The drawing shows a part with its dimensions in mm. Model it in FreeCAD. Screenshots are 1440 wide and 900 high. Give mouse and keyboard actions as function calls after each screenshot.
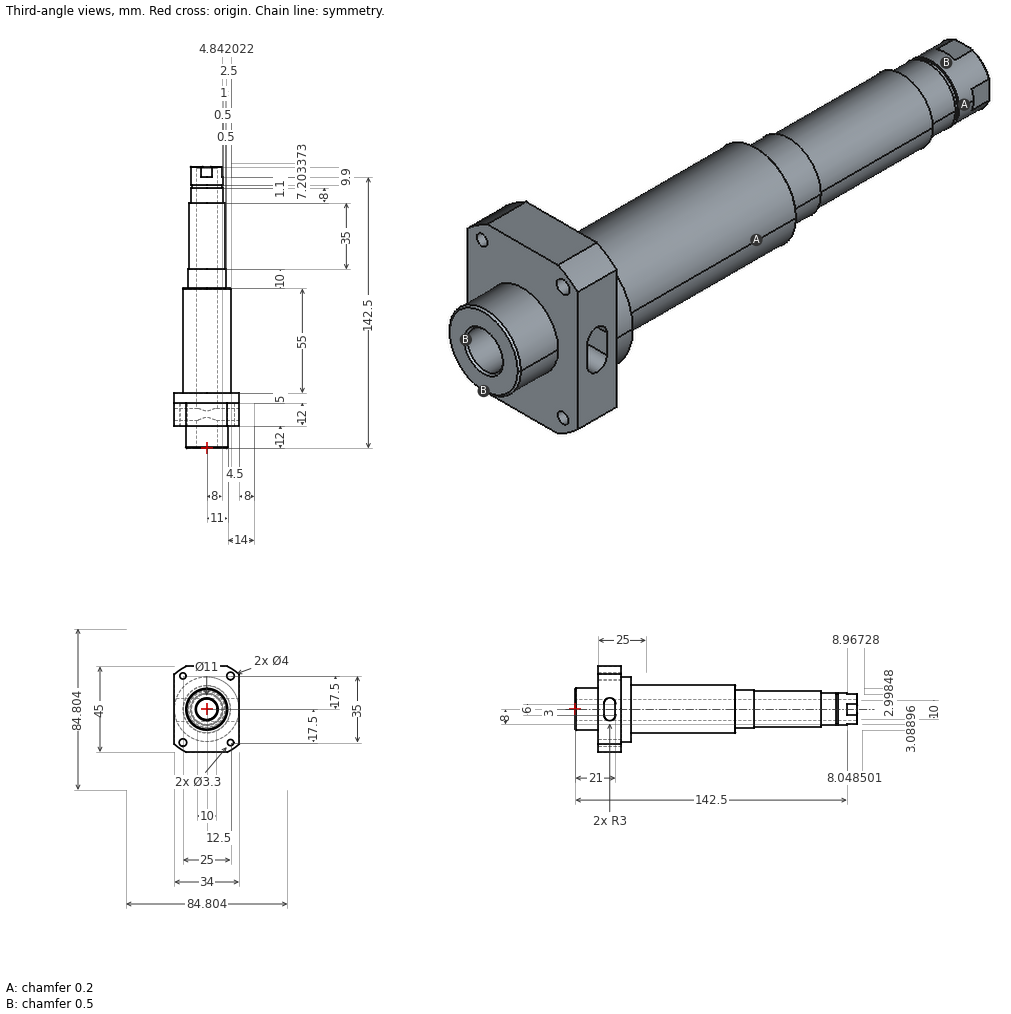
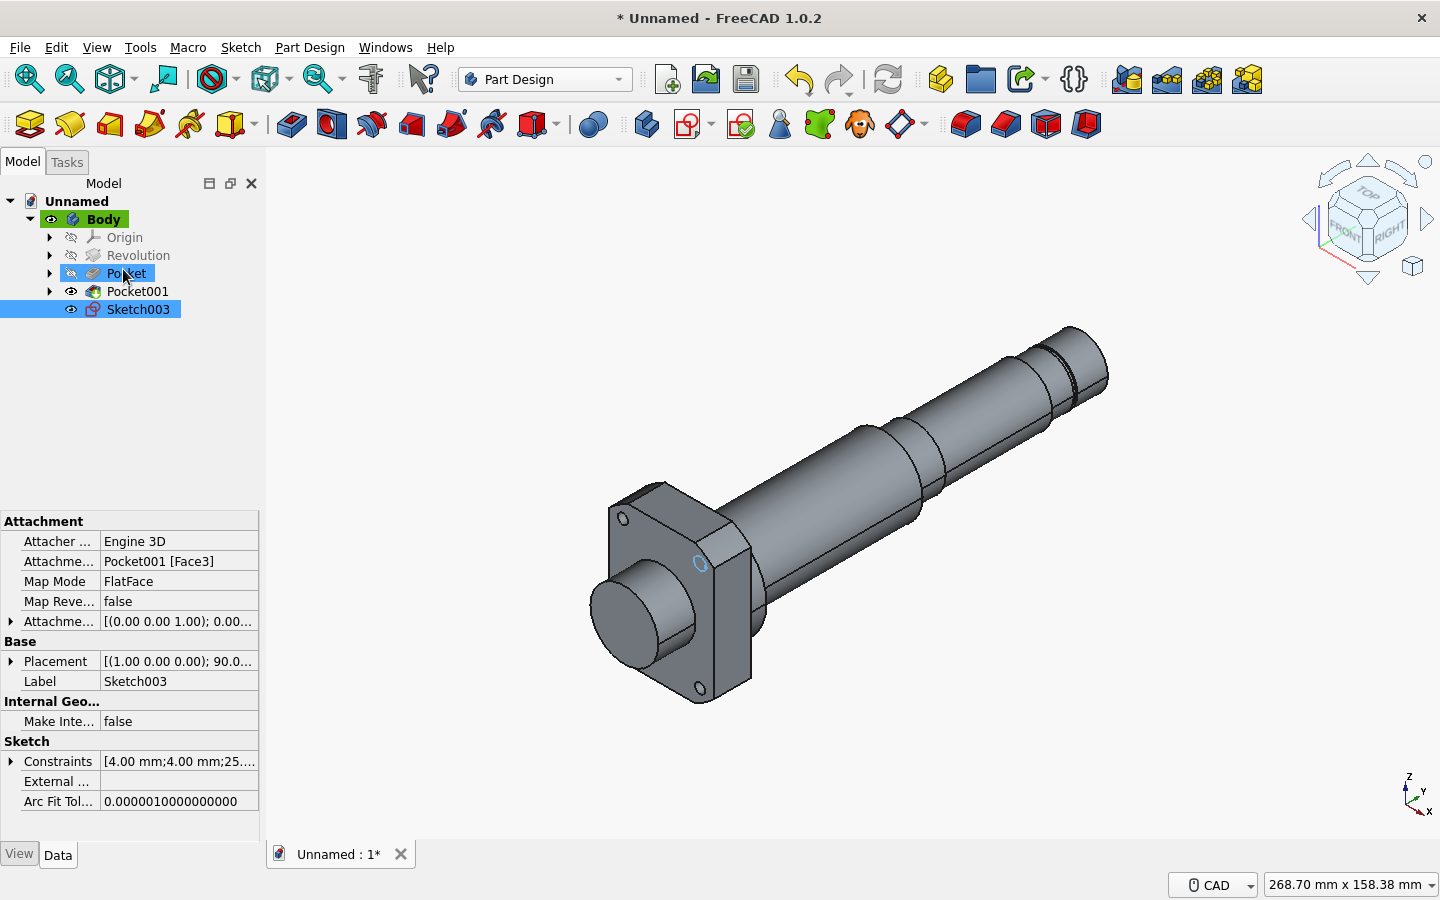
click(292, 124)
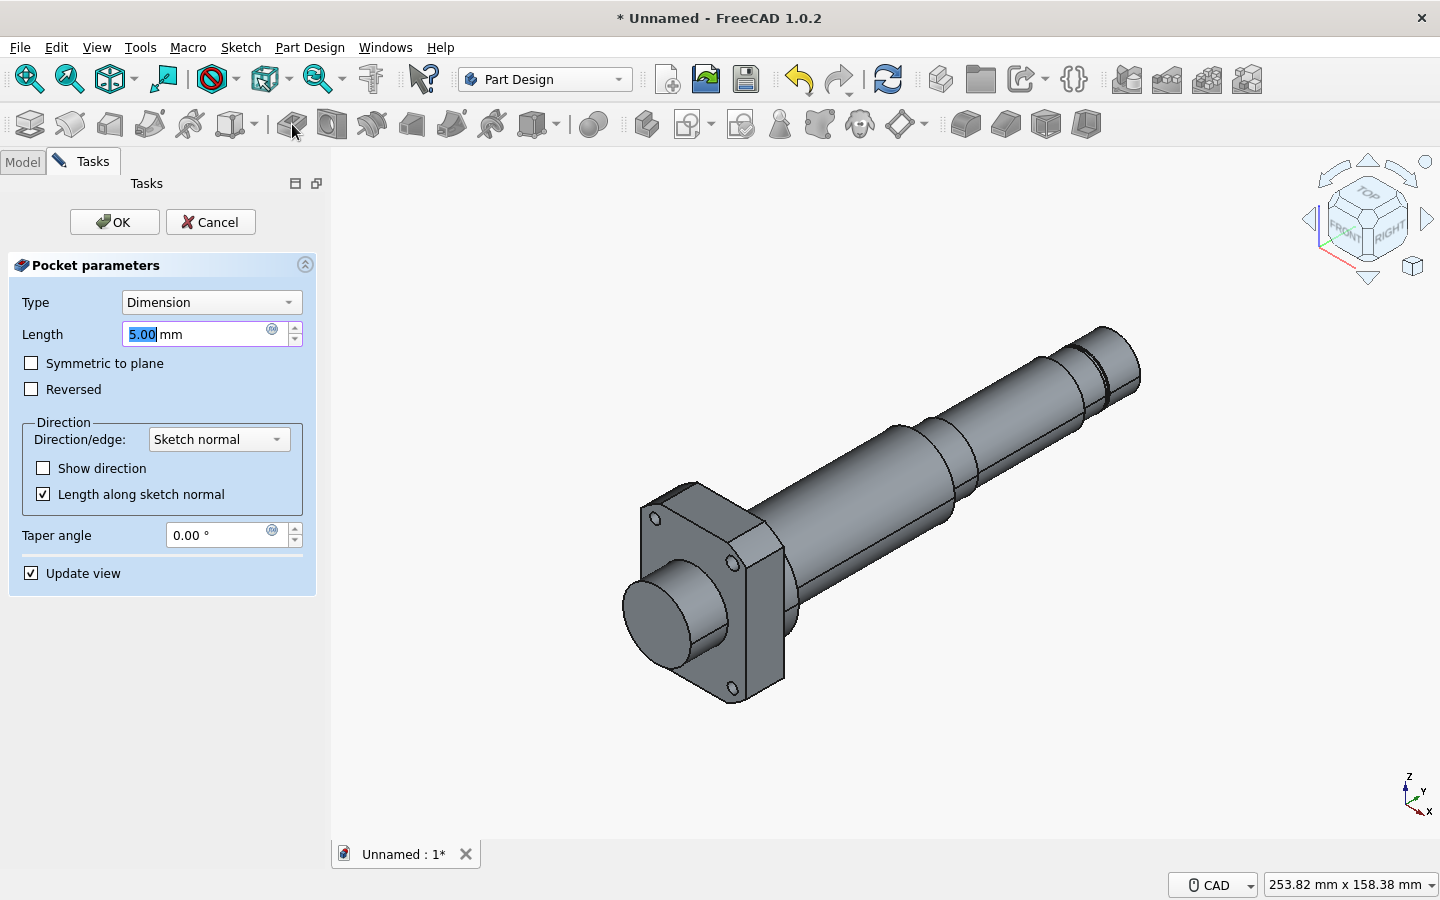
text(25)
key(Tab)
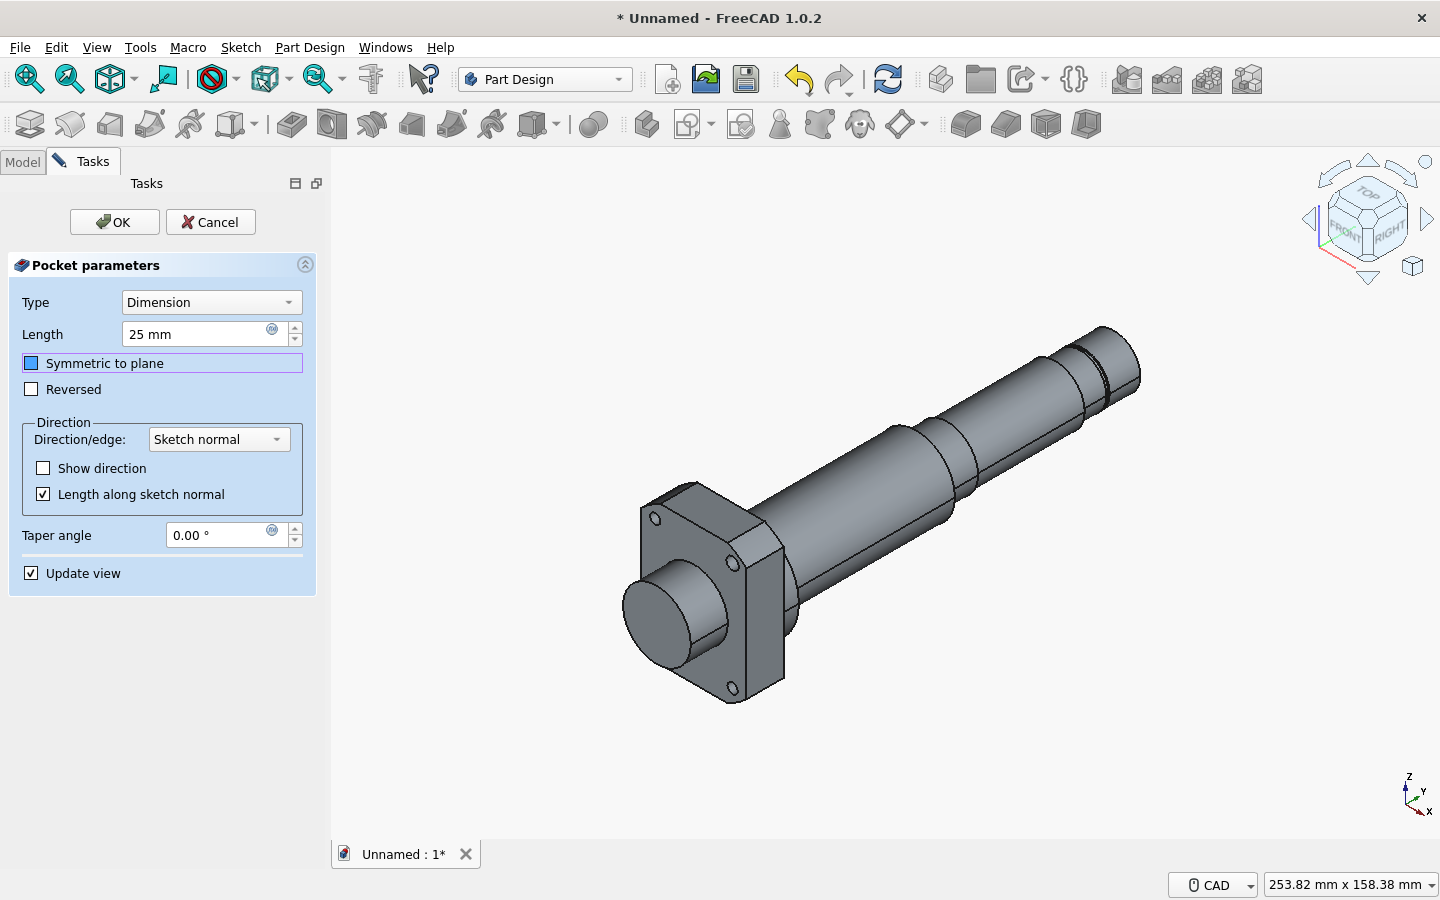
click(115, 222)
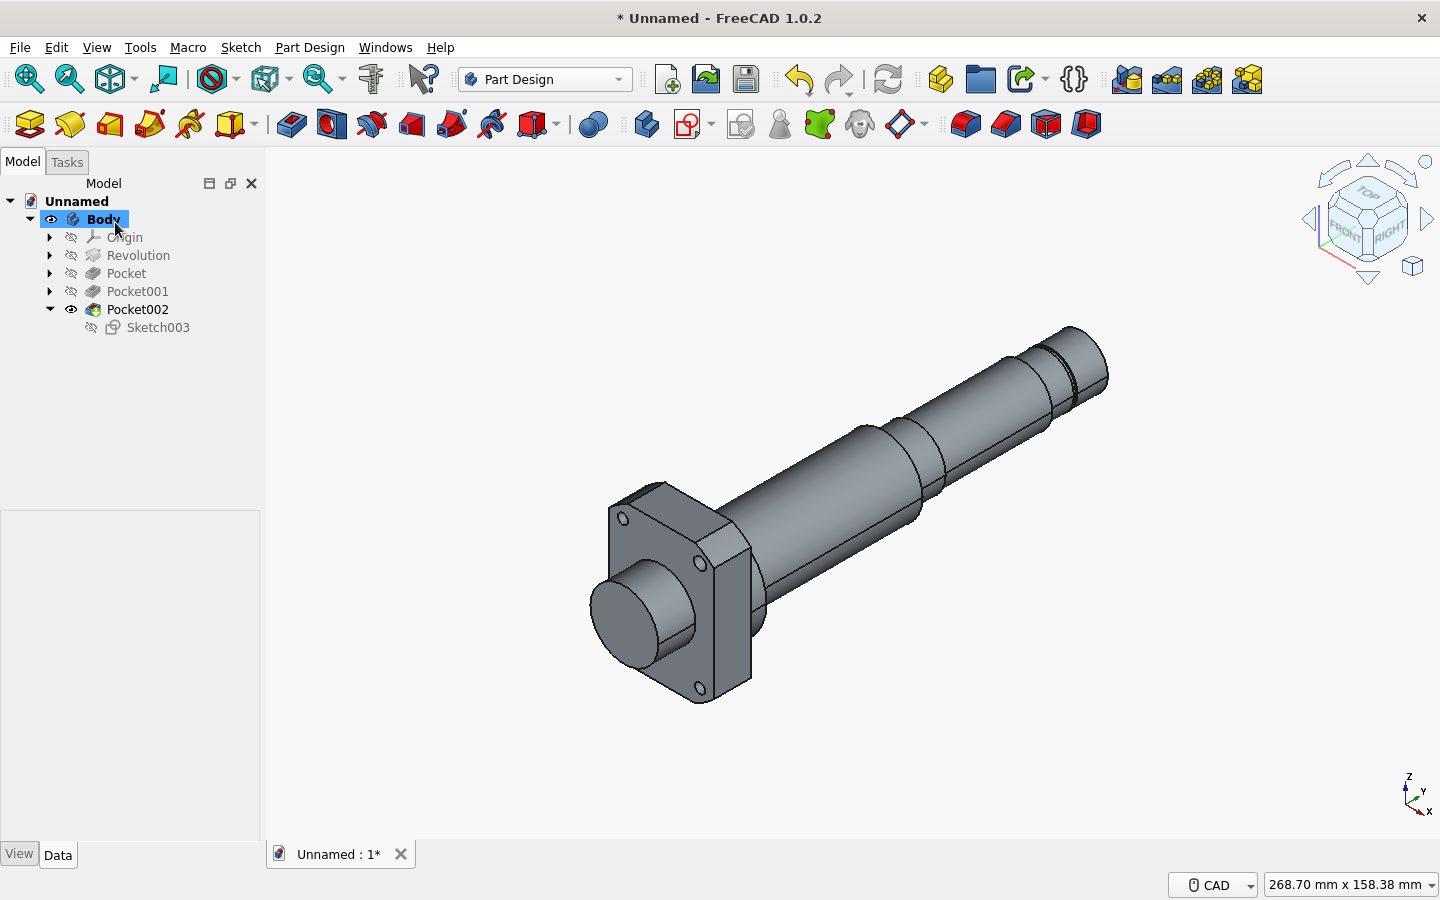
click(688, 124)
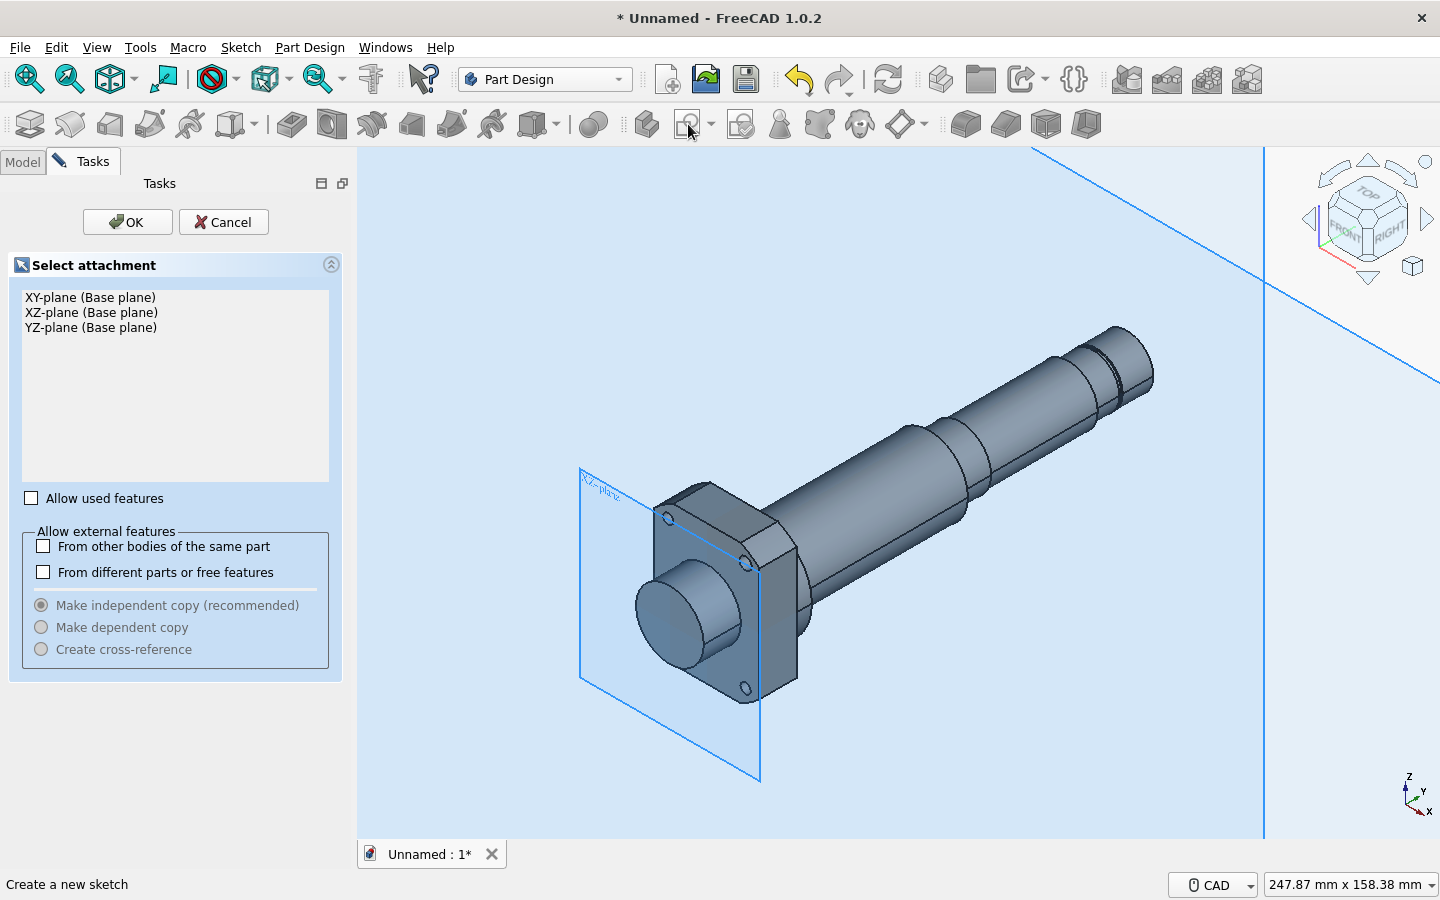
click(82, 312)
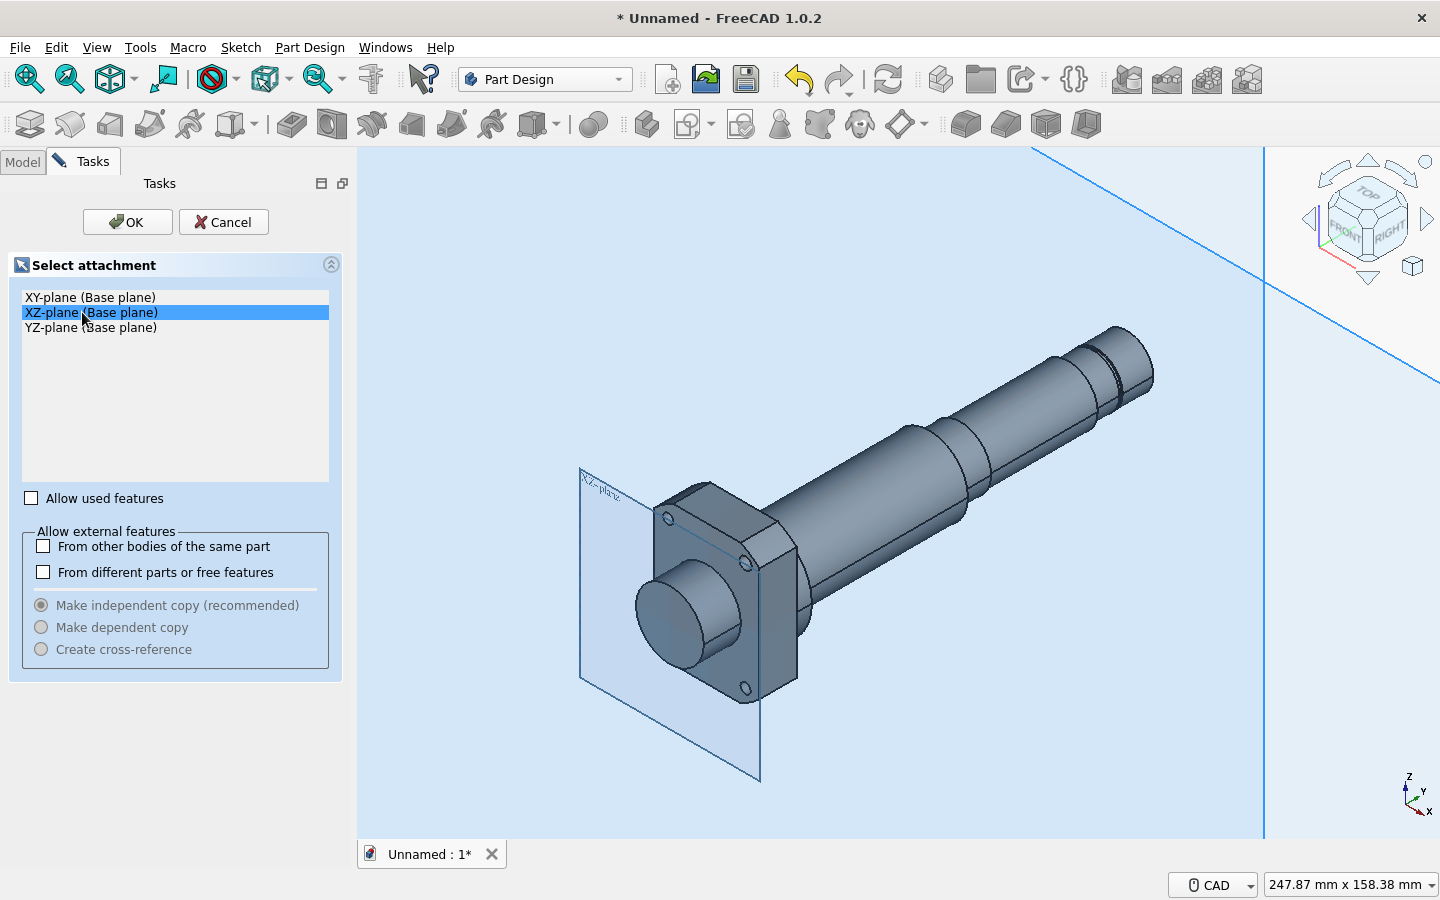
click(128, 222)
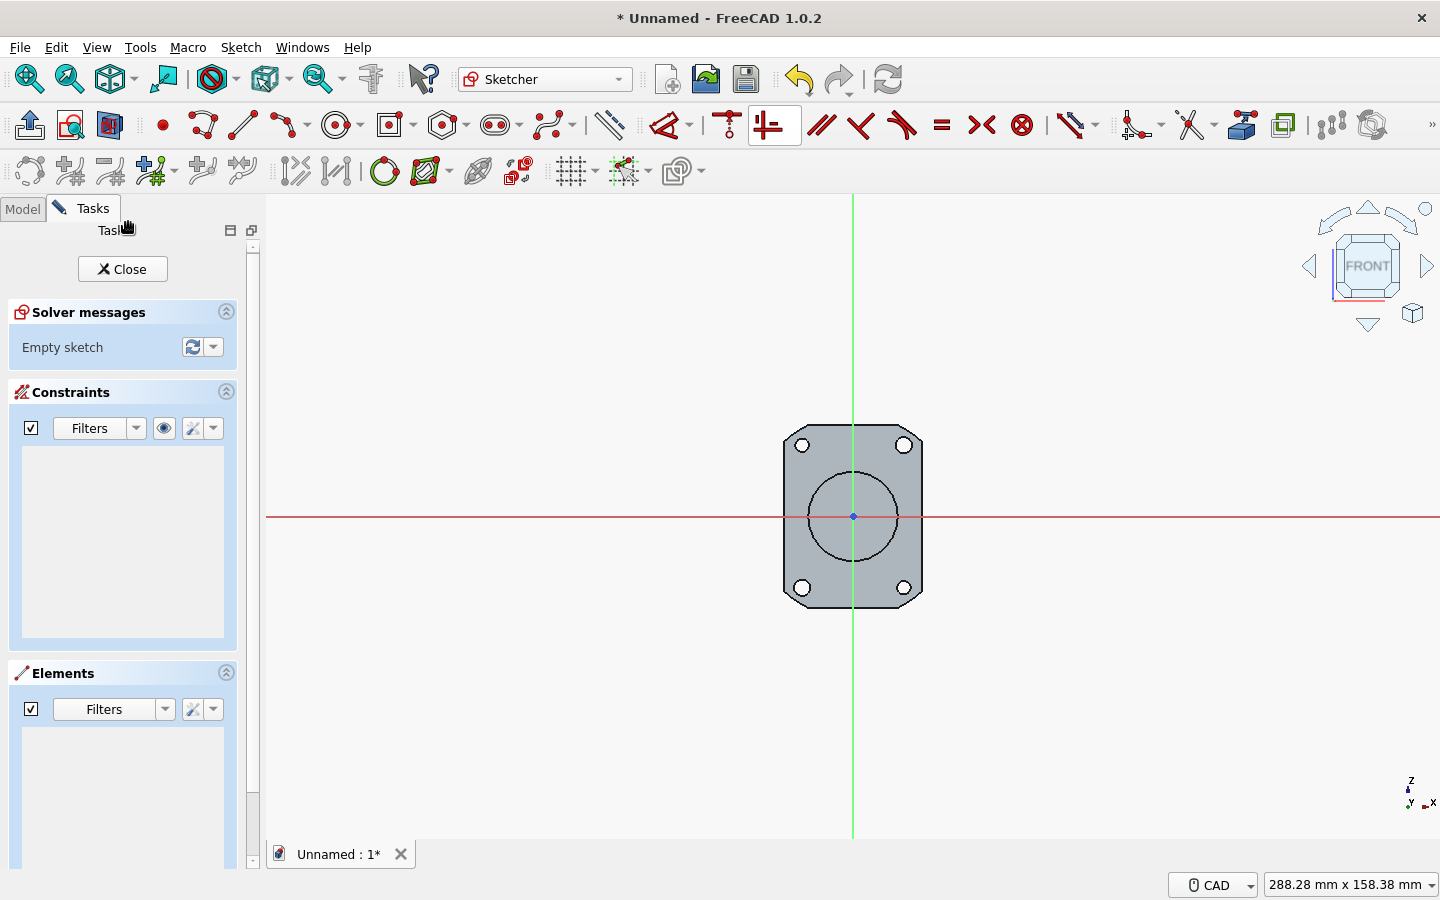
scroll(862, 516, up, 11)